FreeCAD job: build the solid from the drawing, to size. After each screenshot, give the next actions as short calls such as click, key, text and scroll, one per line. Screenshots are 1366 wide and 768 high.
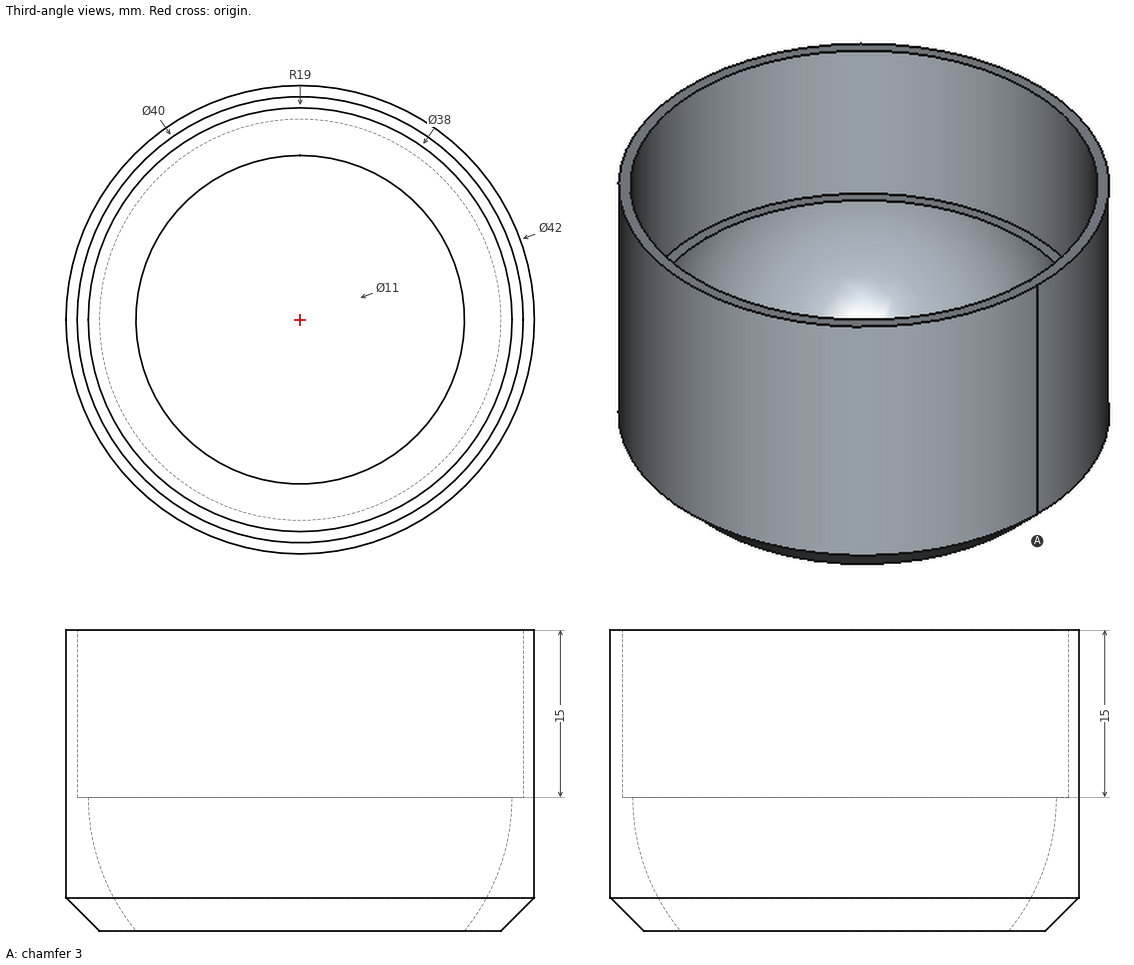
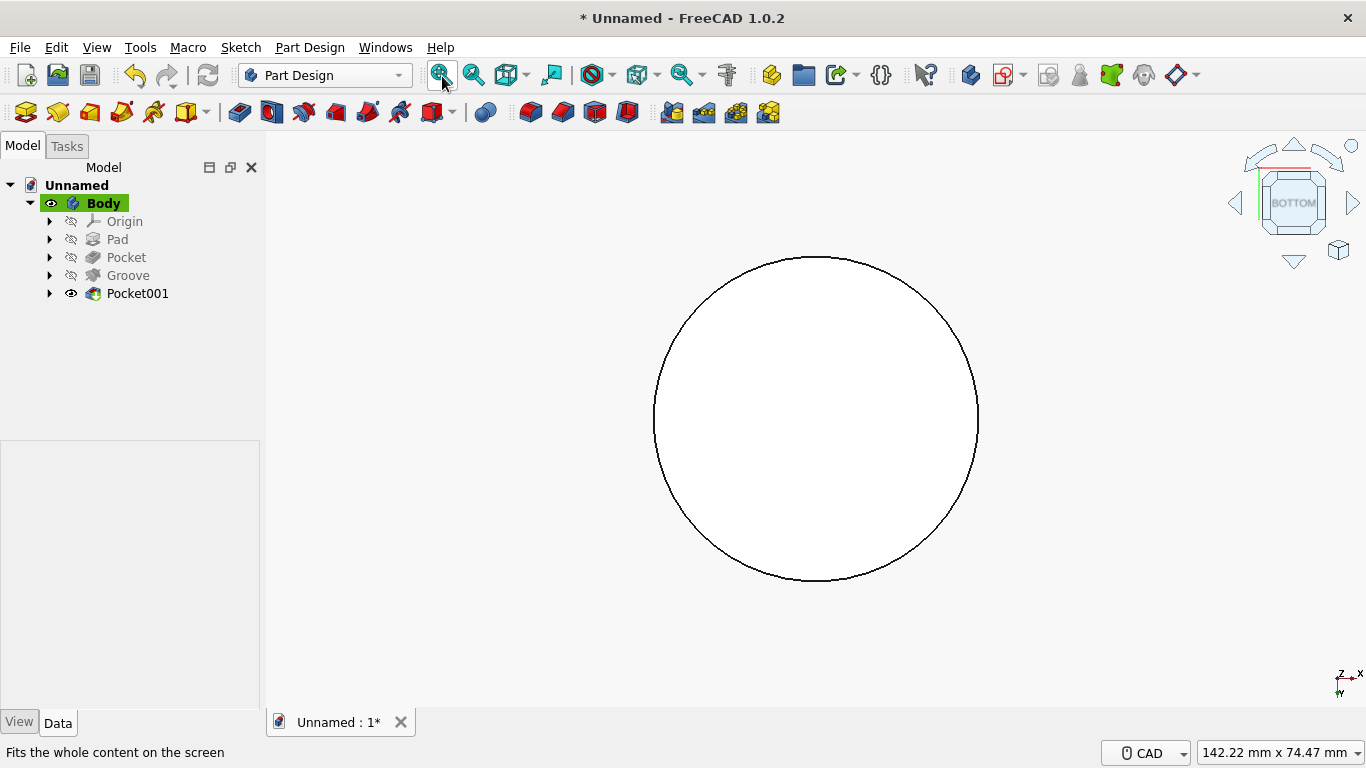
click(816, 418)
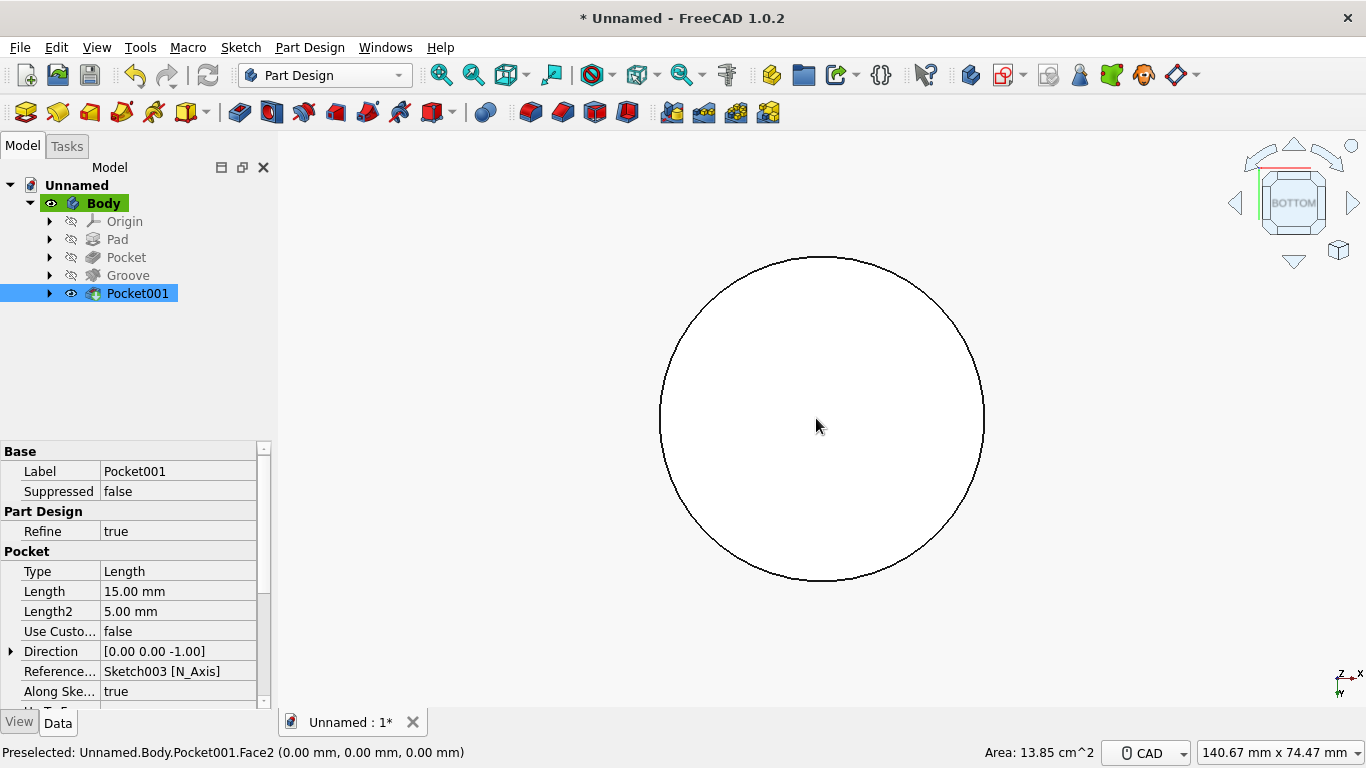
click(1004, 76)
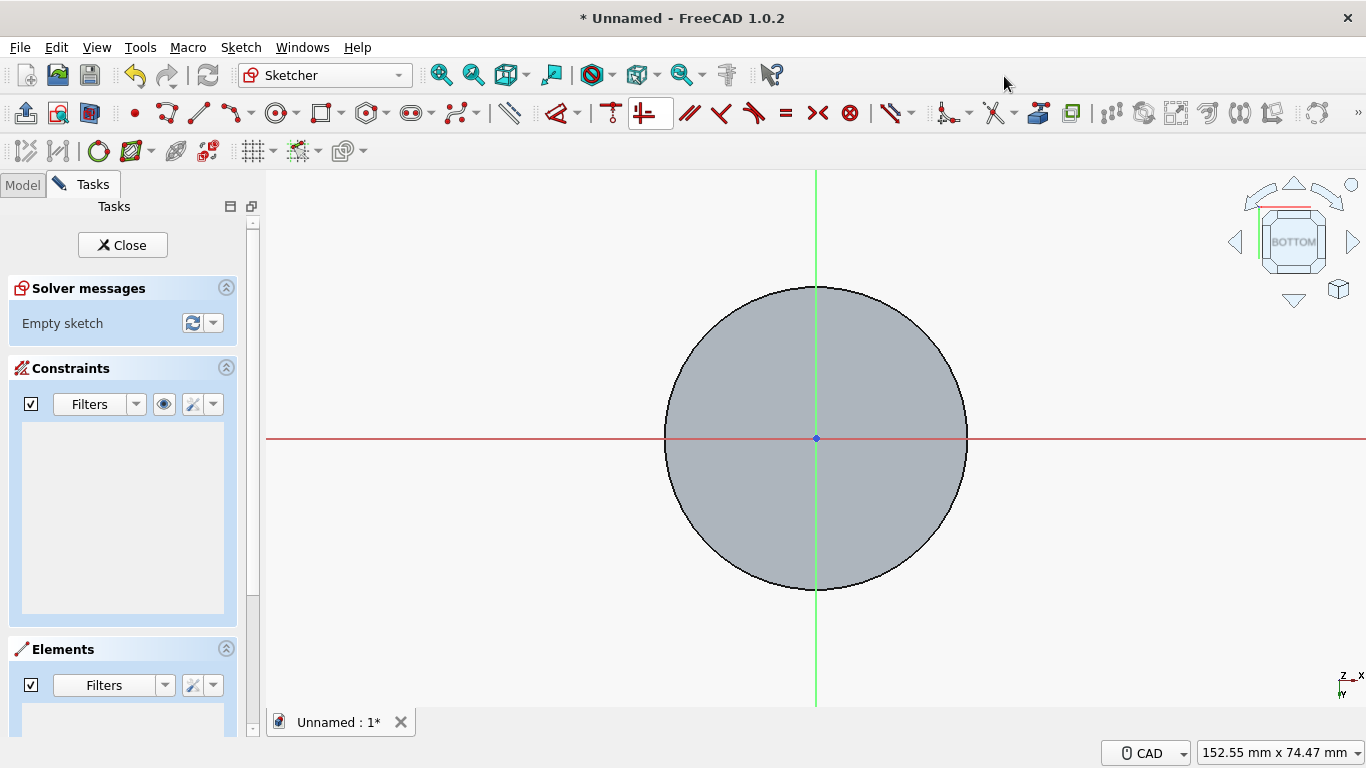
scroll(838, 438, up, 7)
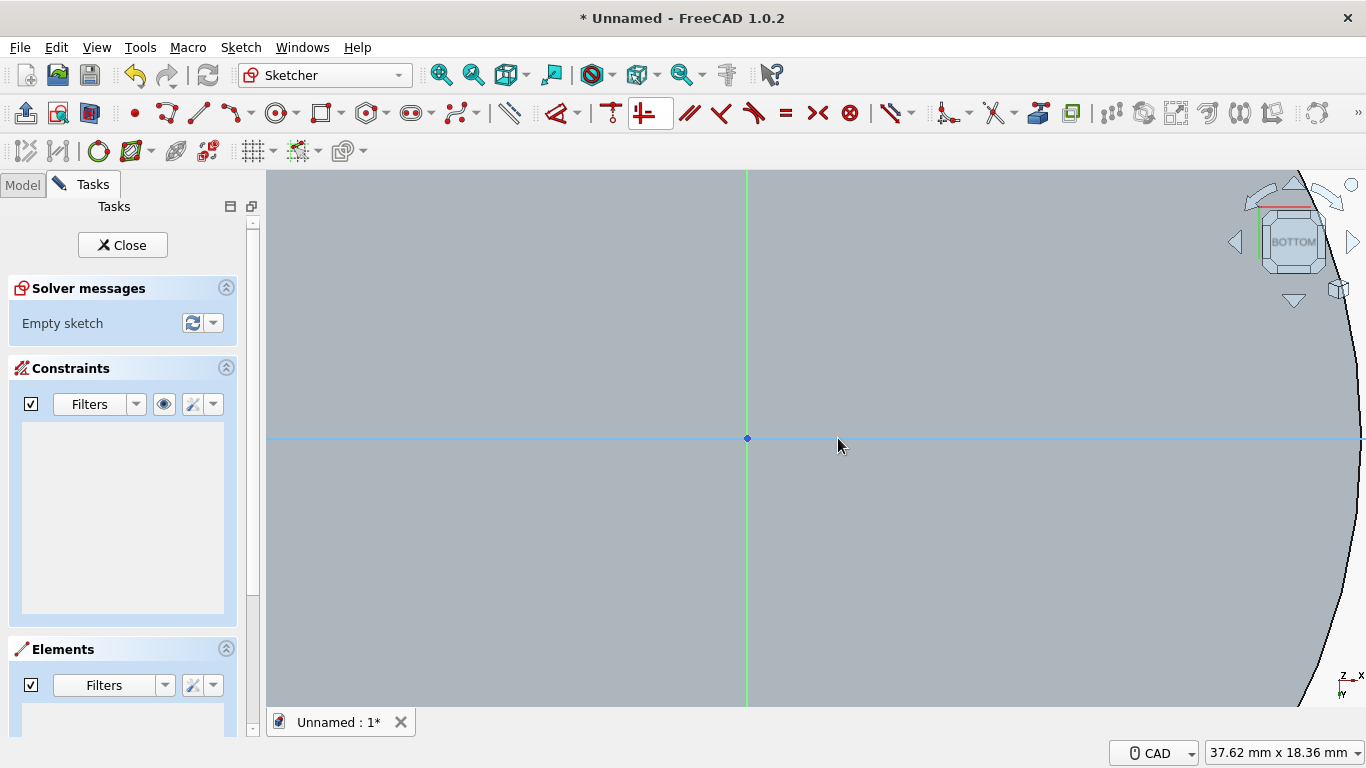
click(276, 114)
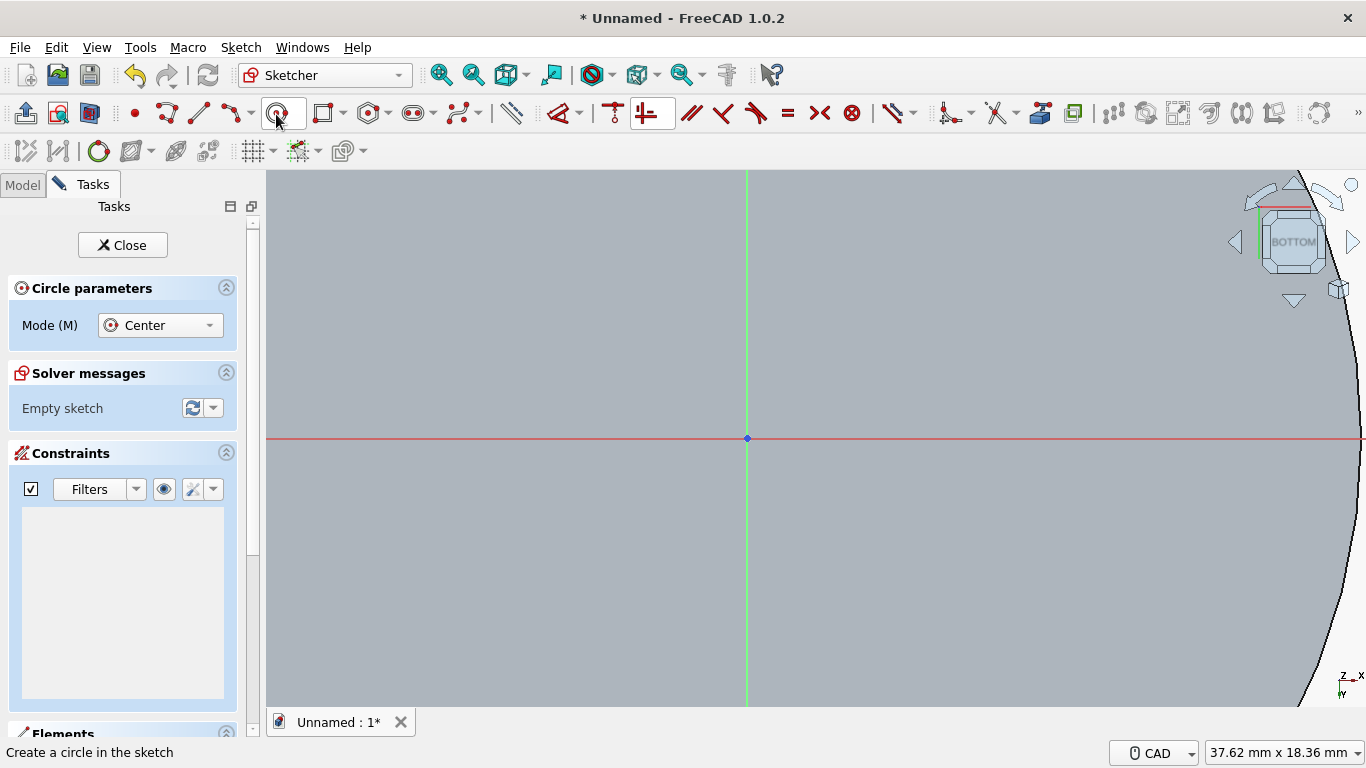
click(747, 438)
move(861, 325)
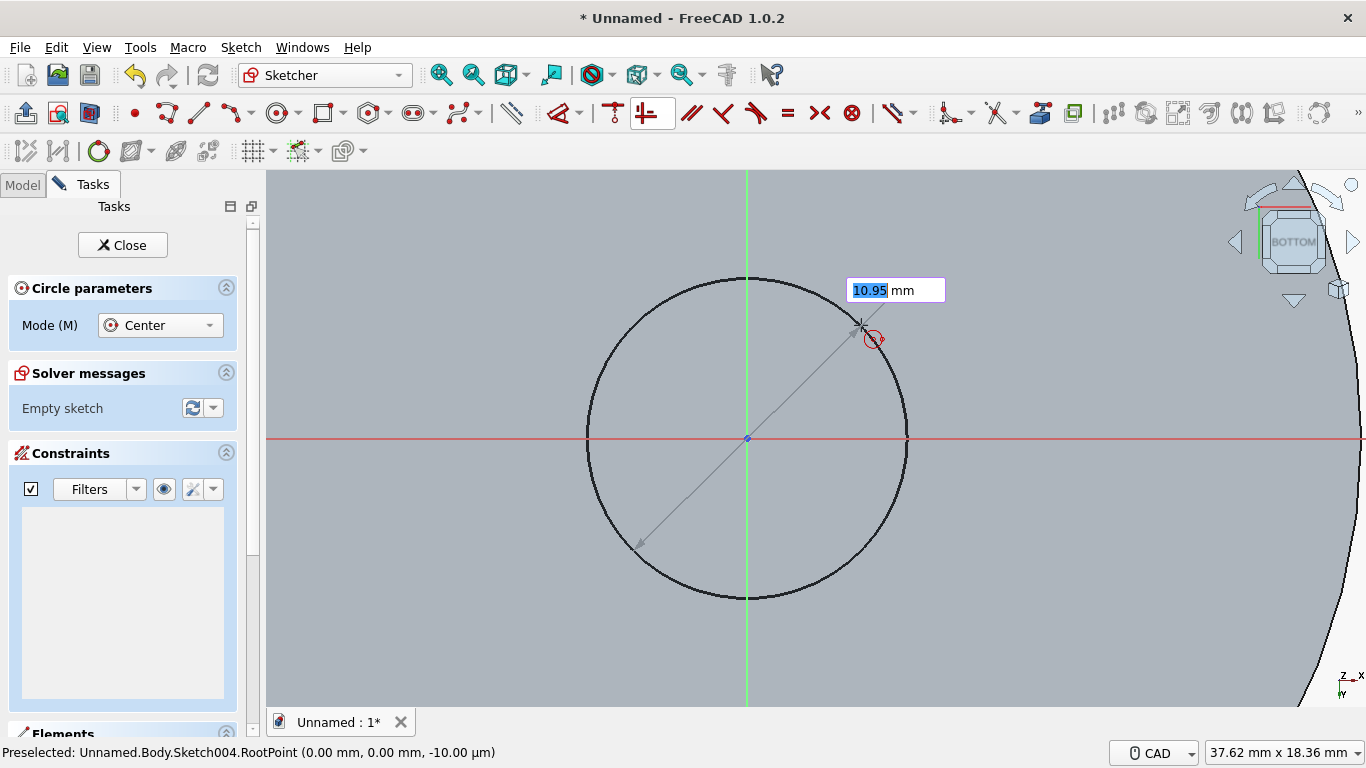
text(11)
key(Return)
key(Escape)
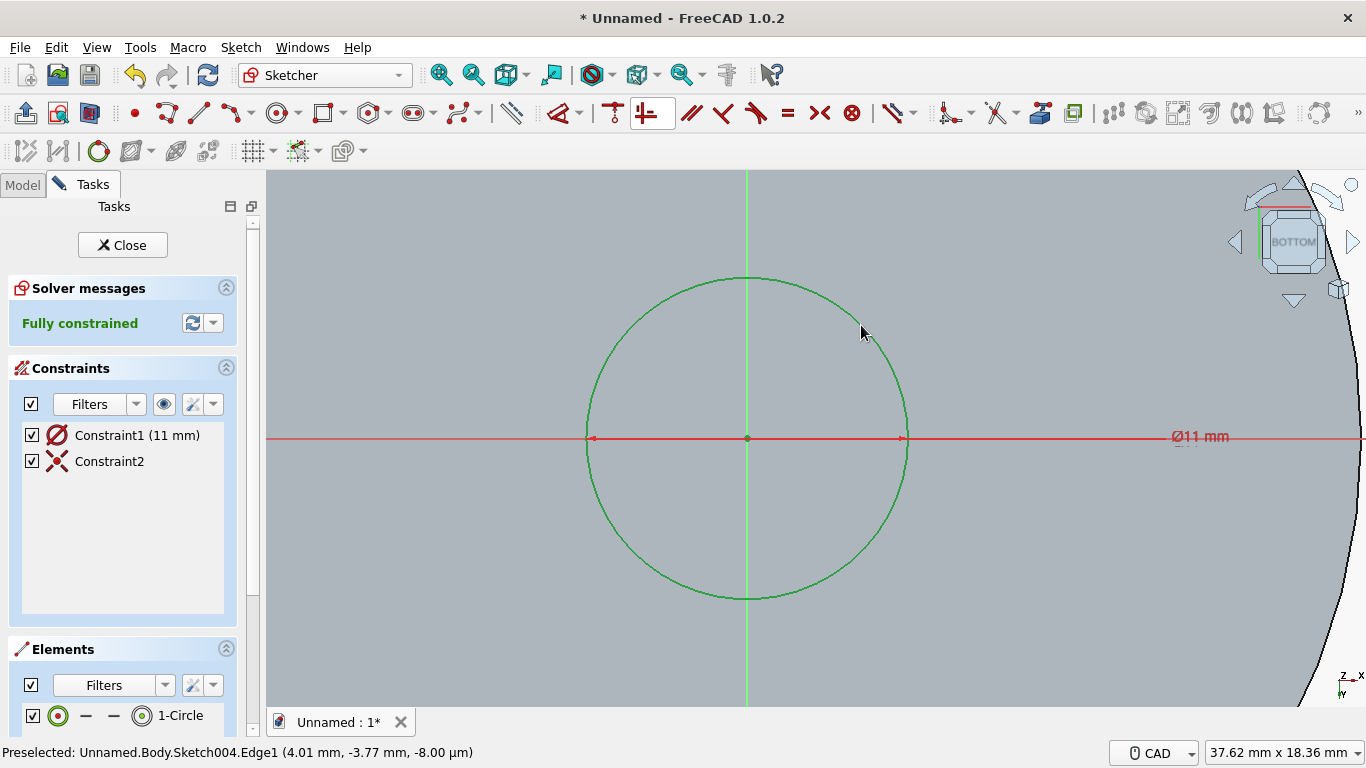
click(123, 245)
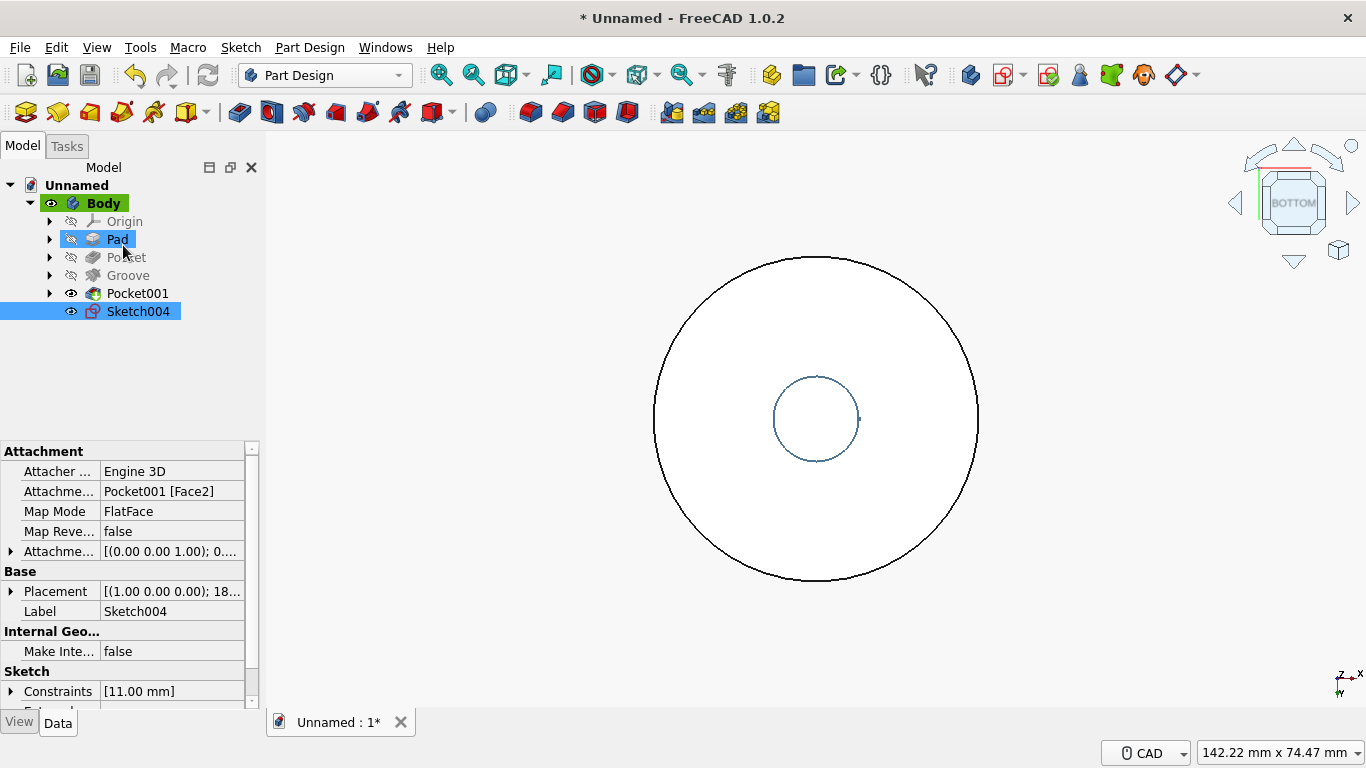
click(240, 112)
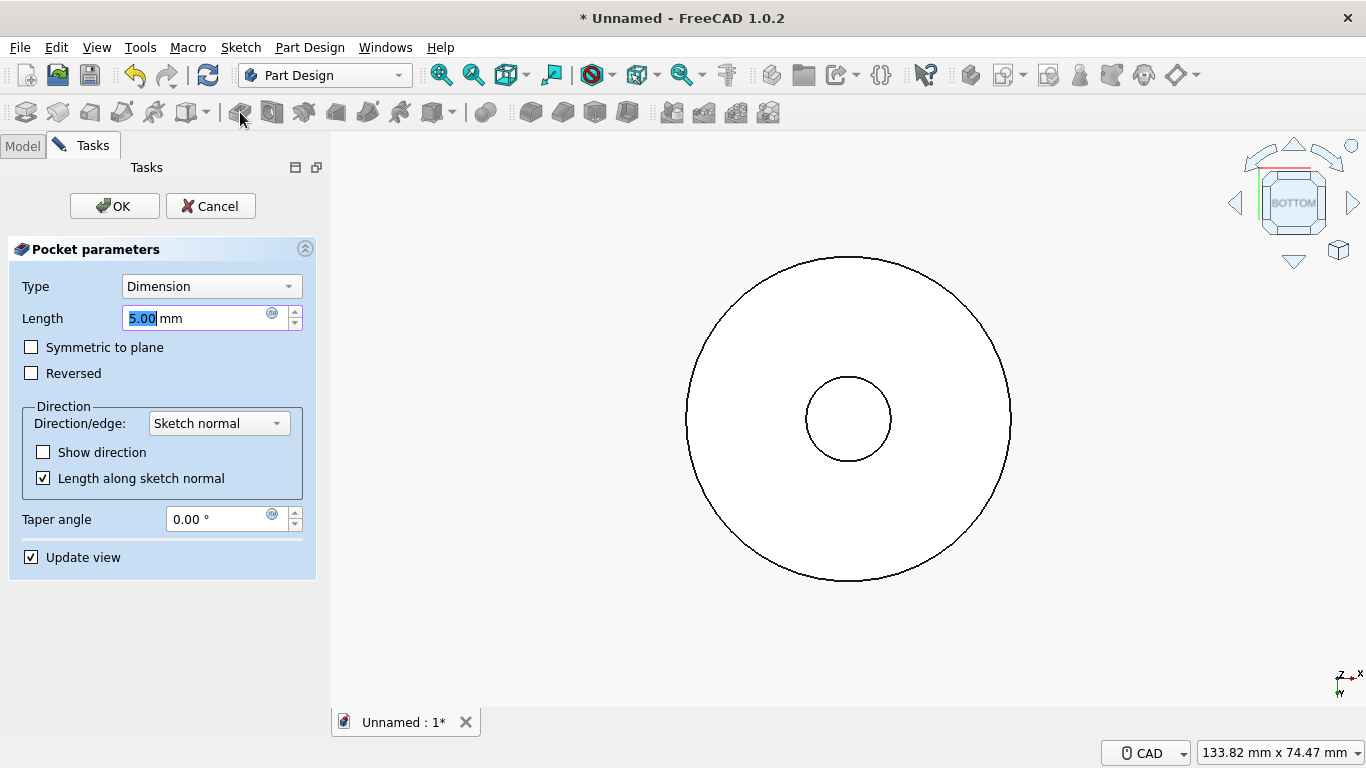
click(212, 286)